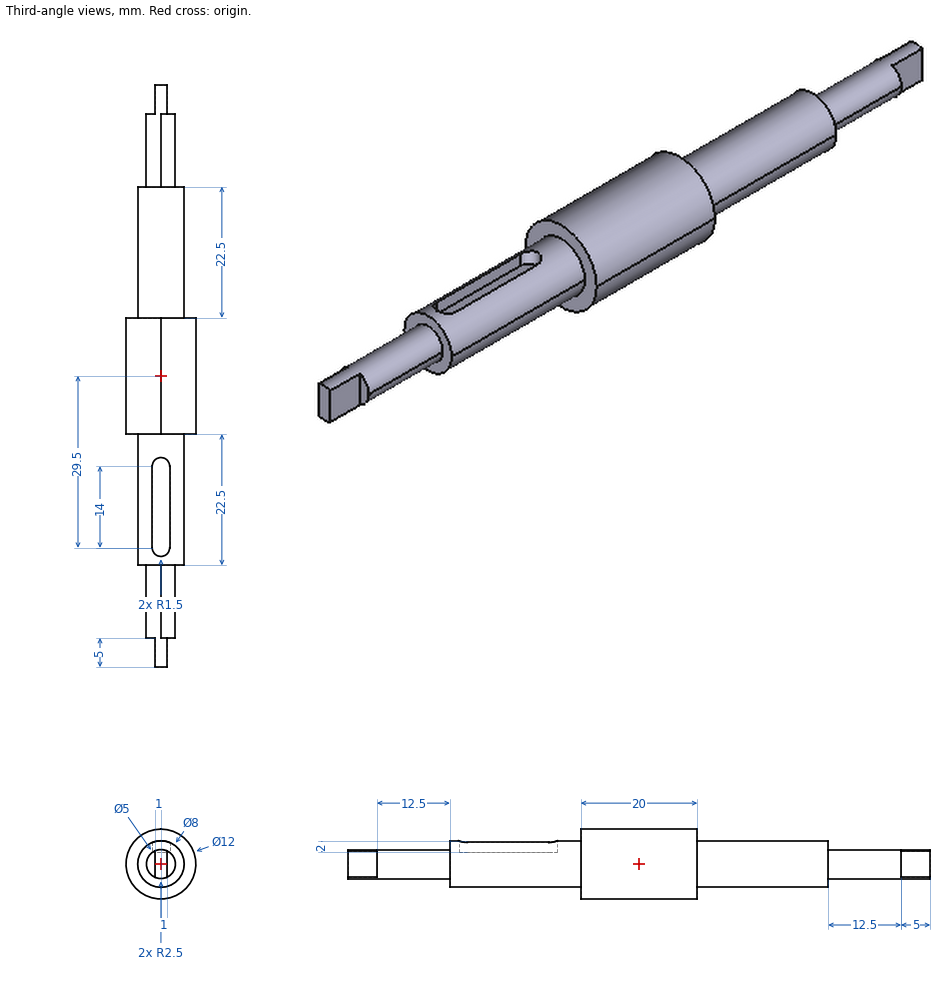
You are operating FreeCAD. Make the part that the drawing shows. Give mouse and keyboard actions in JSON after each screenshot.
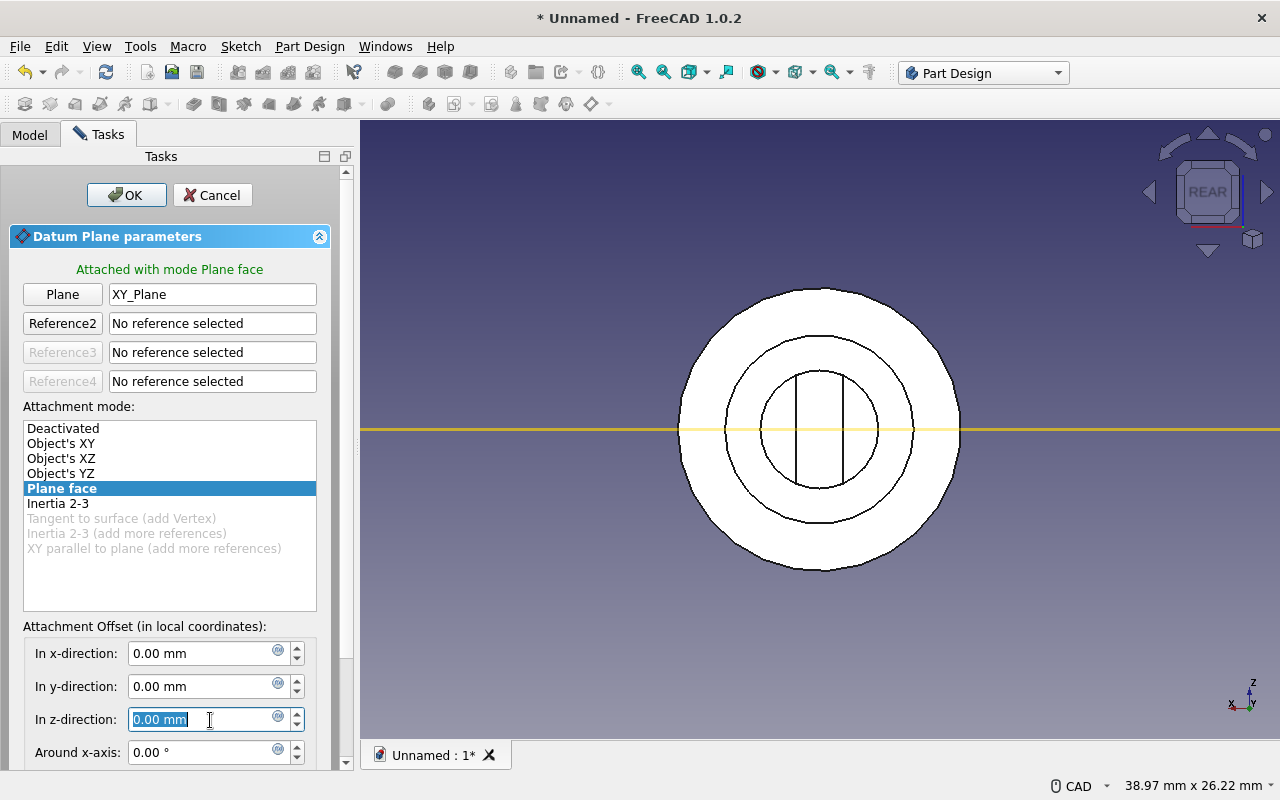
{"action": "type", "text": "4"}
{"action": "key", "text": "Tab"}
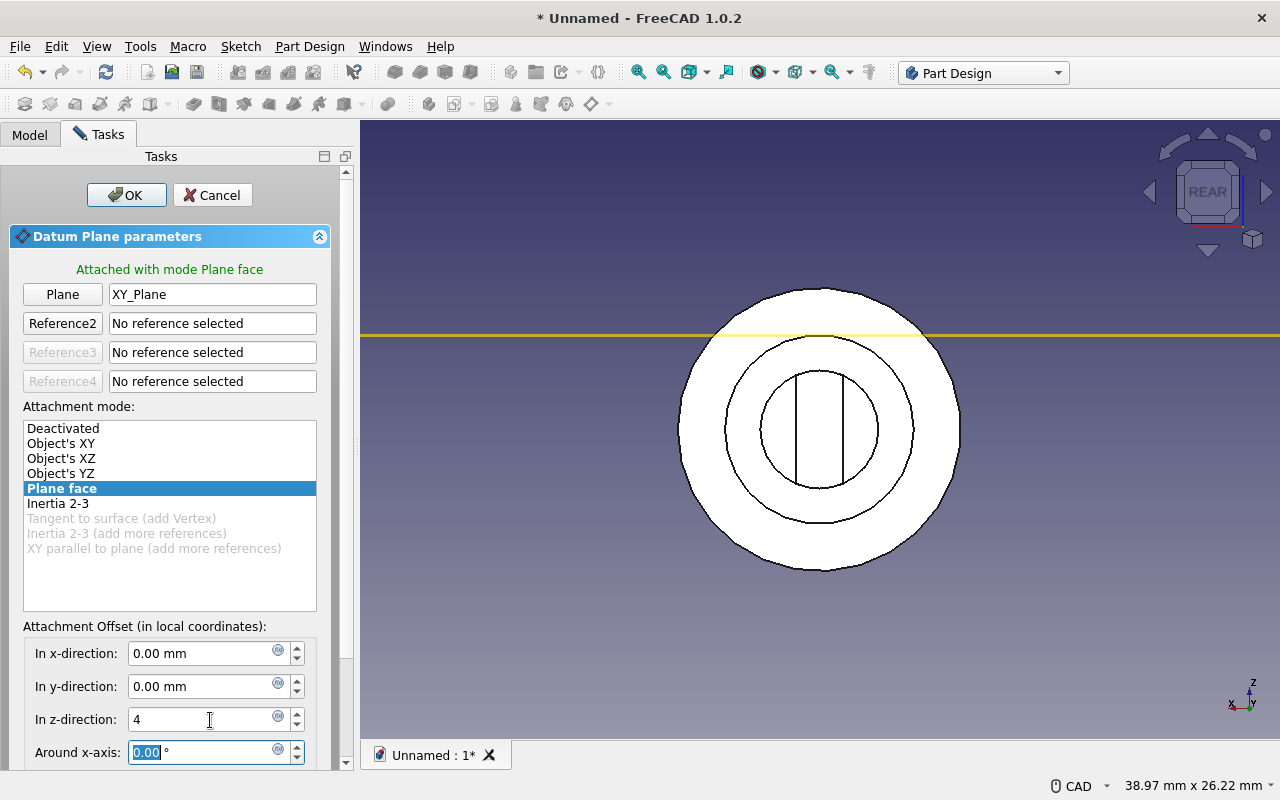
{"action": "left_click", "coordinate": [127, 195]}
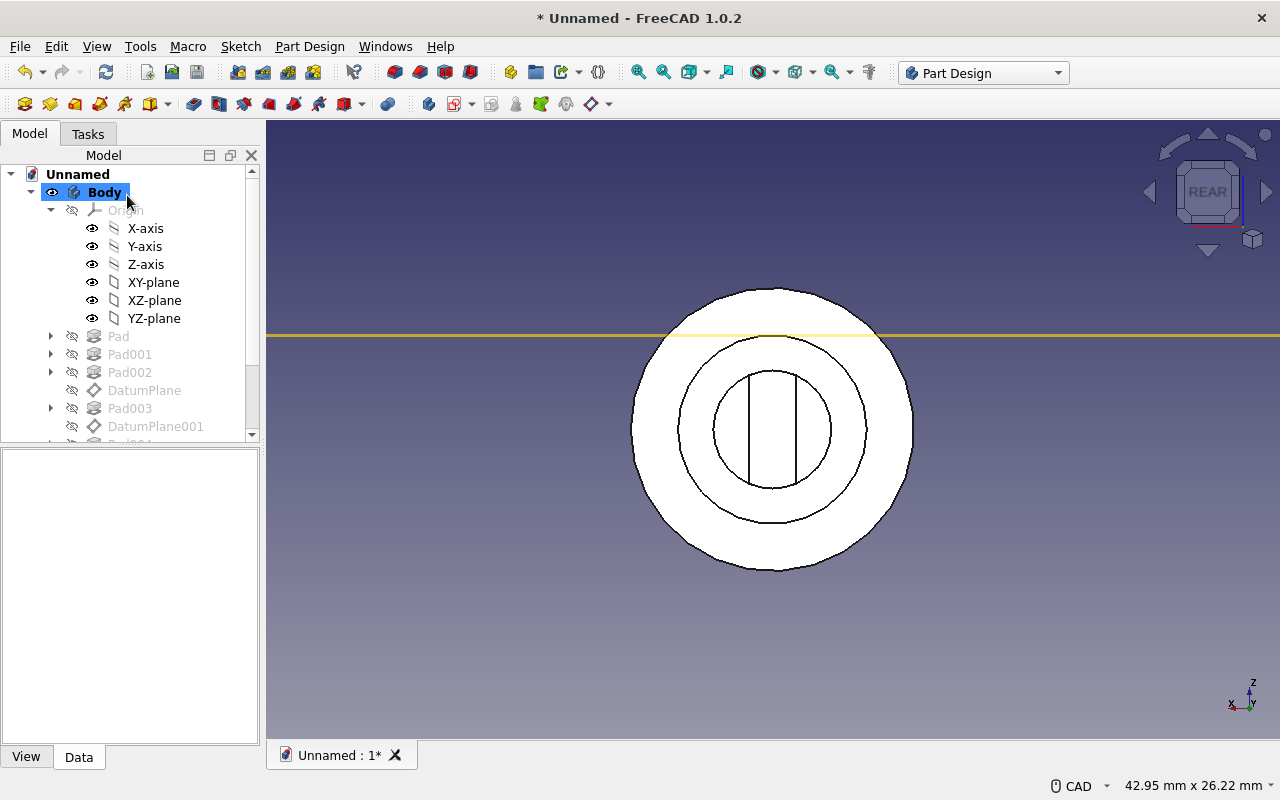
{"action": "scroll", "coordinate": [101, 296], "scroll_direction": "down", "scroll_amount": 3}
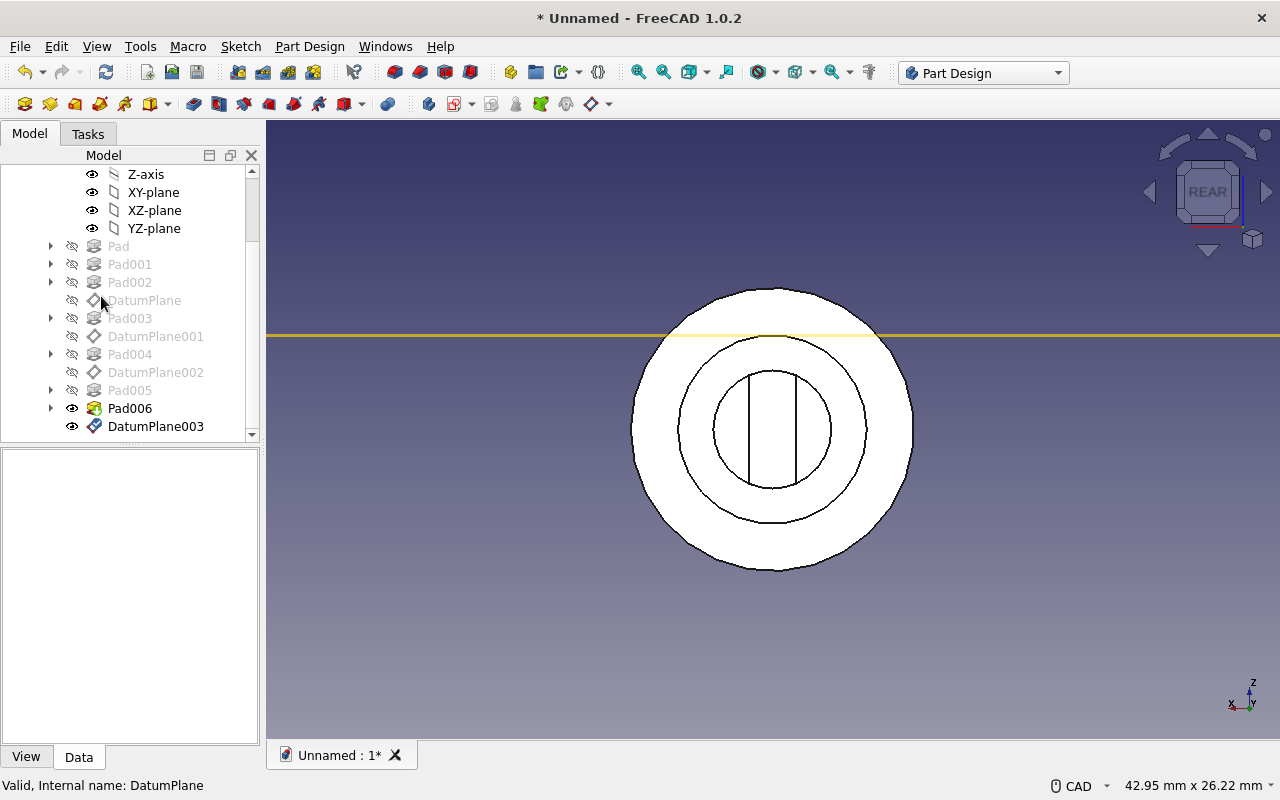
{"action": "left_click", "coordinate": [117, 426]}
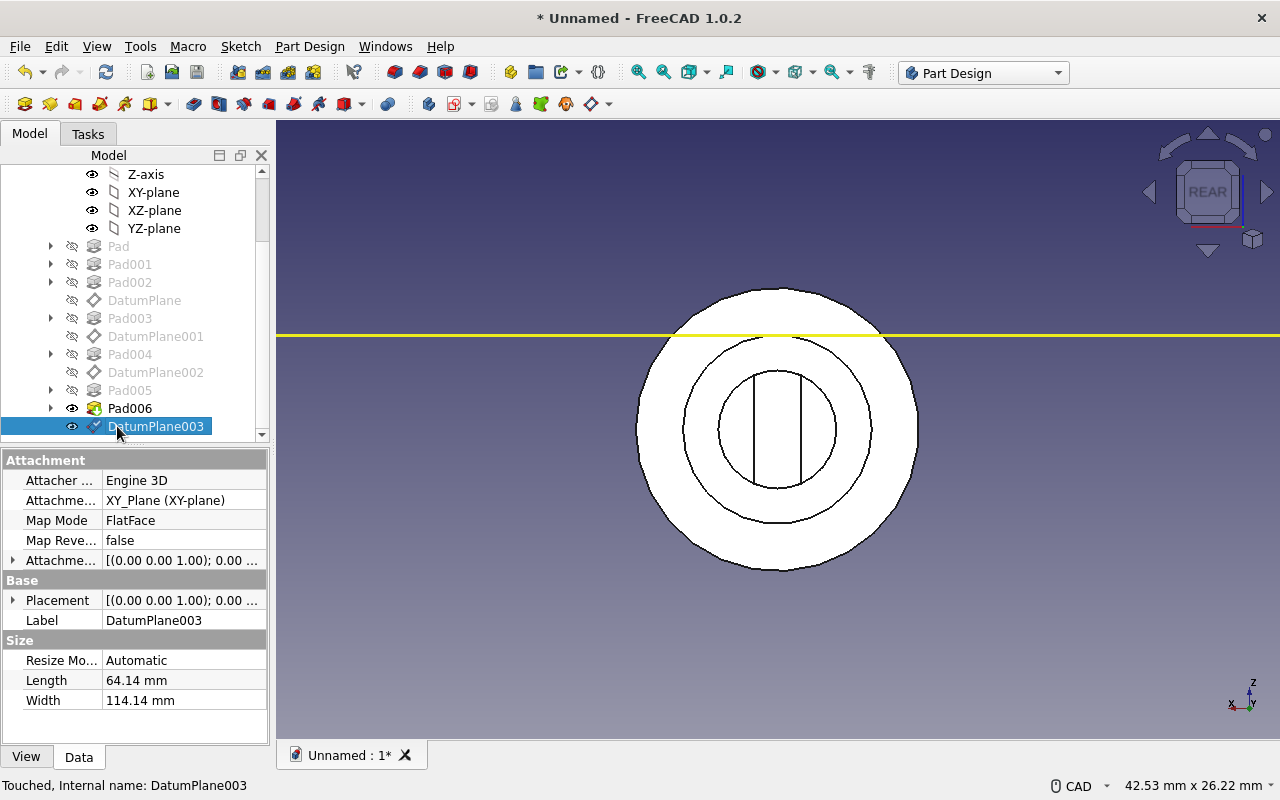
{"action": "left_click", "coordinate": [454, 104]}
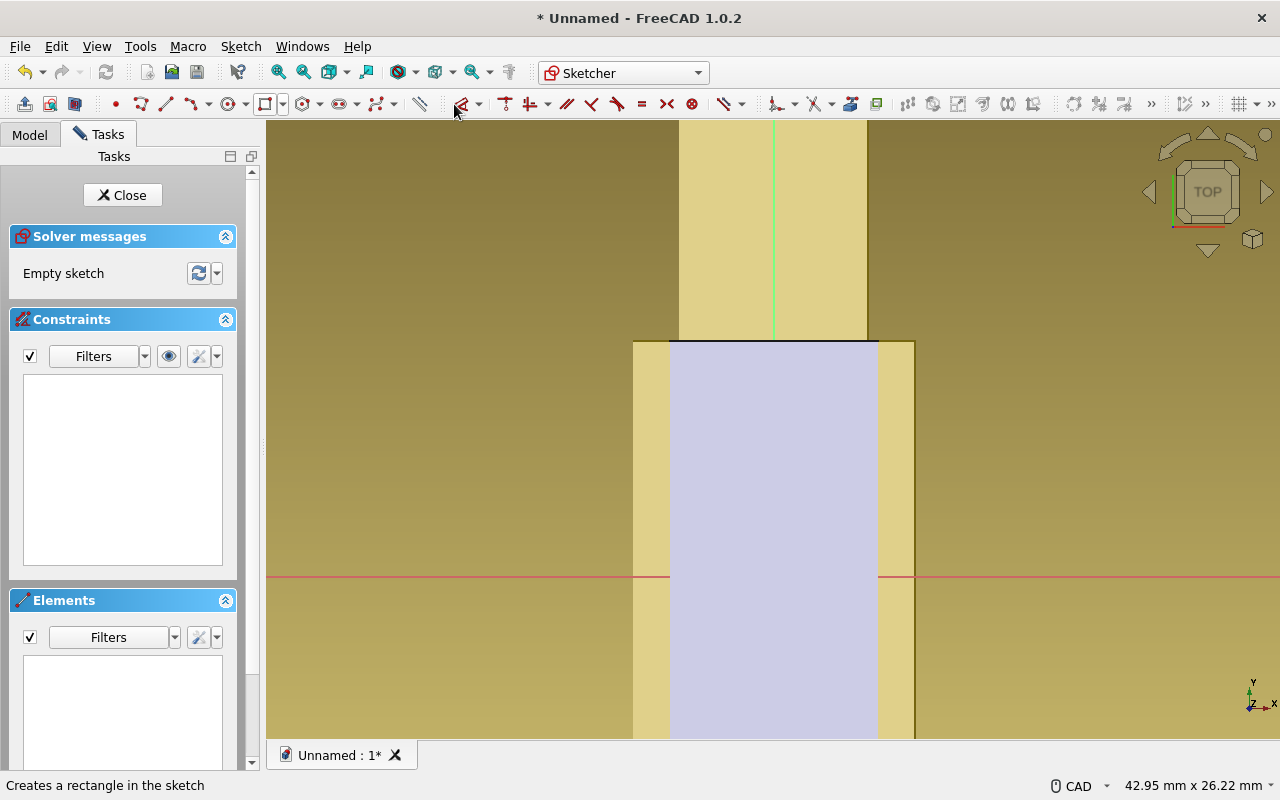
{"action": "left_click", "coordinate": [75, 104]}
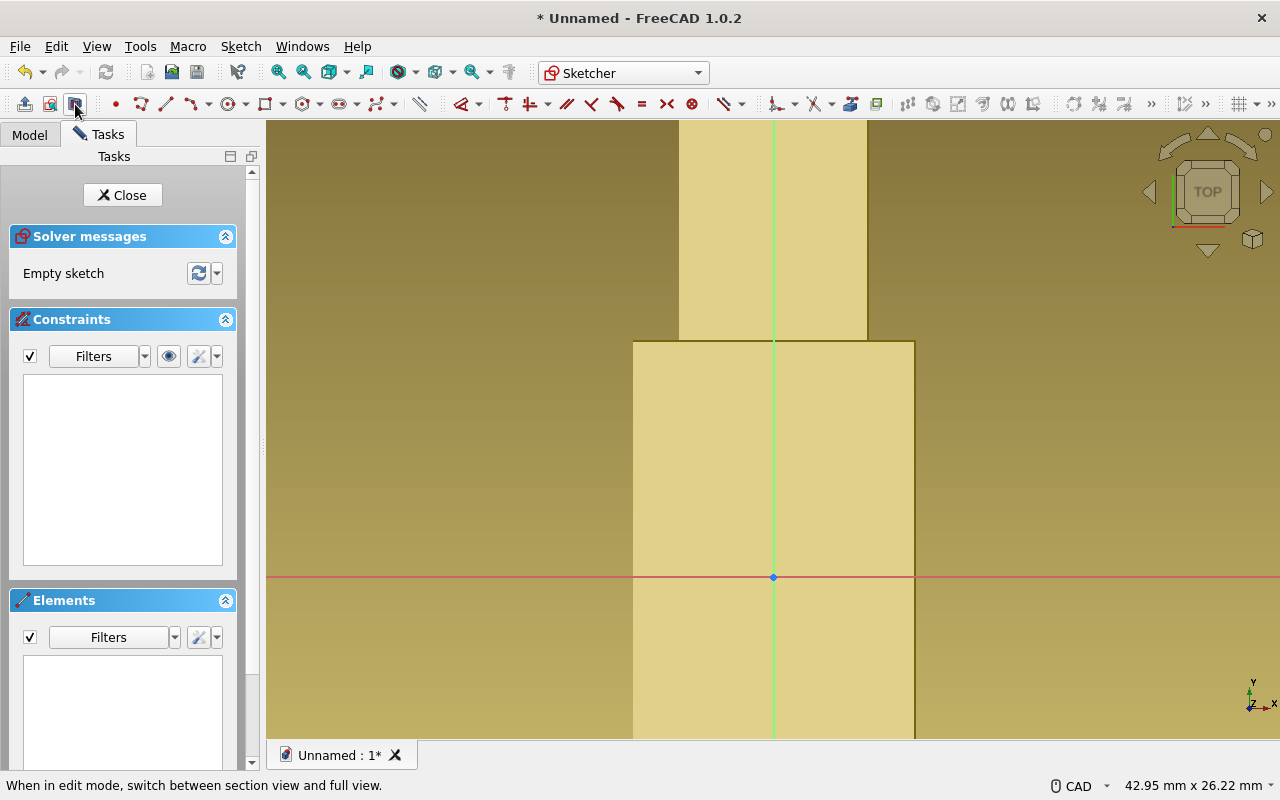
{"action": "scroll", "coordinate": [648, 148], "scroll_direction": "down", "scroll_amount": 4}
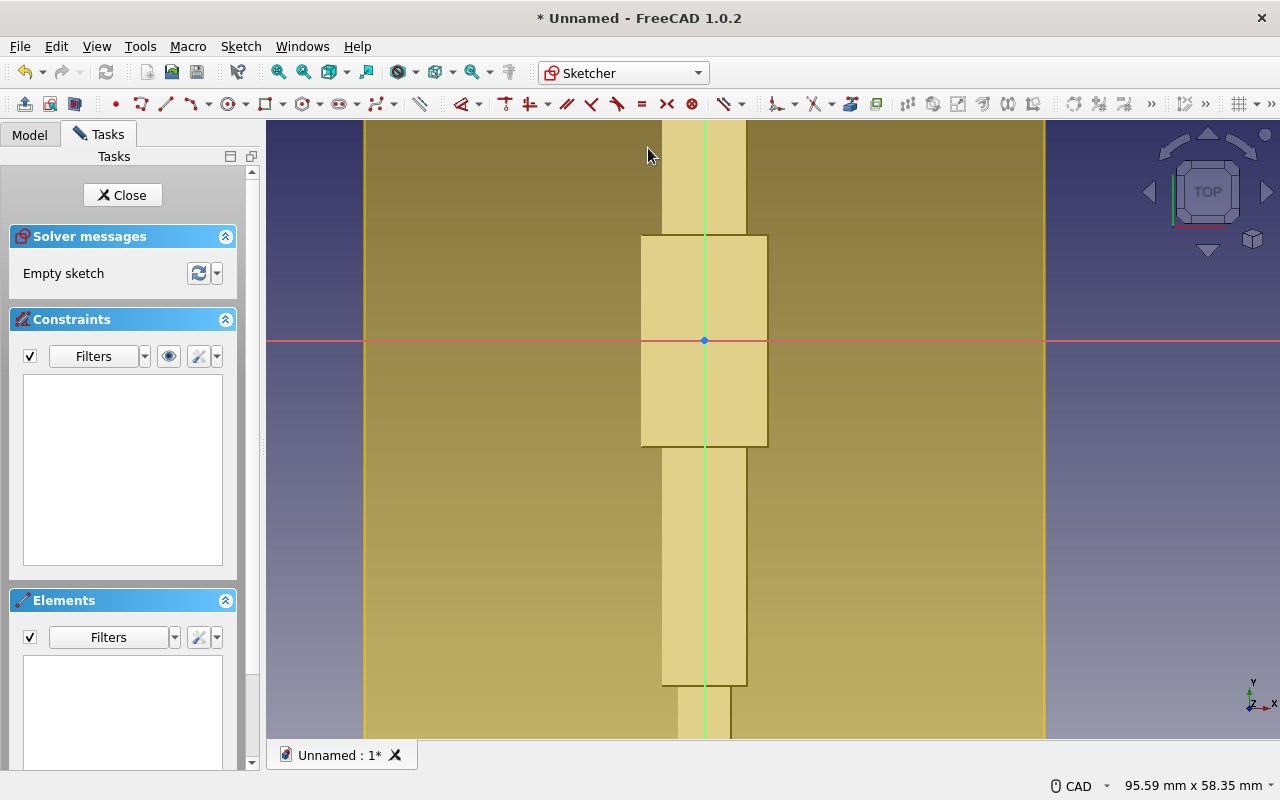
{"action": "key", "text": "g s"}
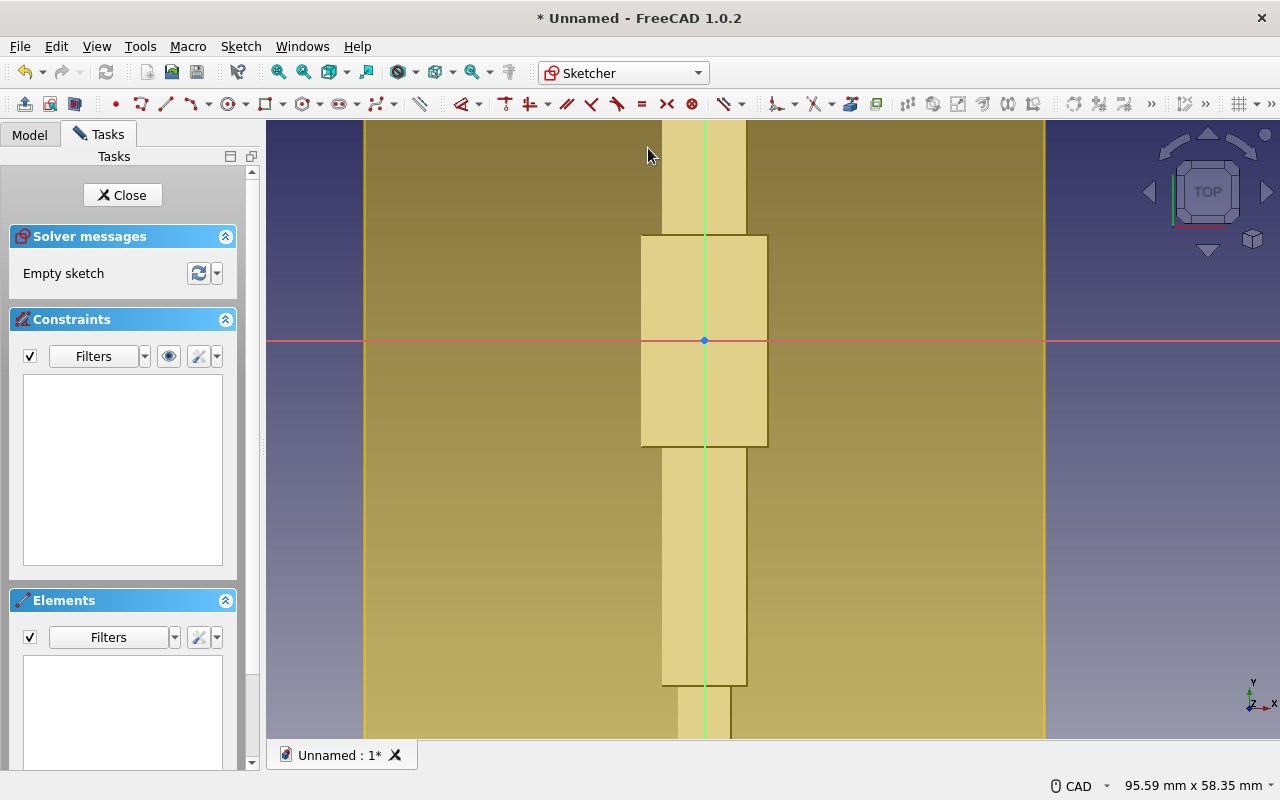
{"action": "scroll", "coordinate": [705, 654], "scroll_direction": "up", "scroll_amount": 2}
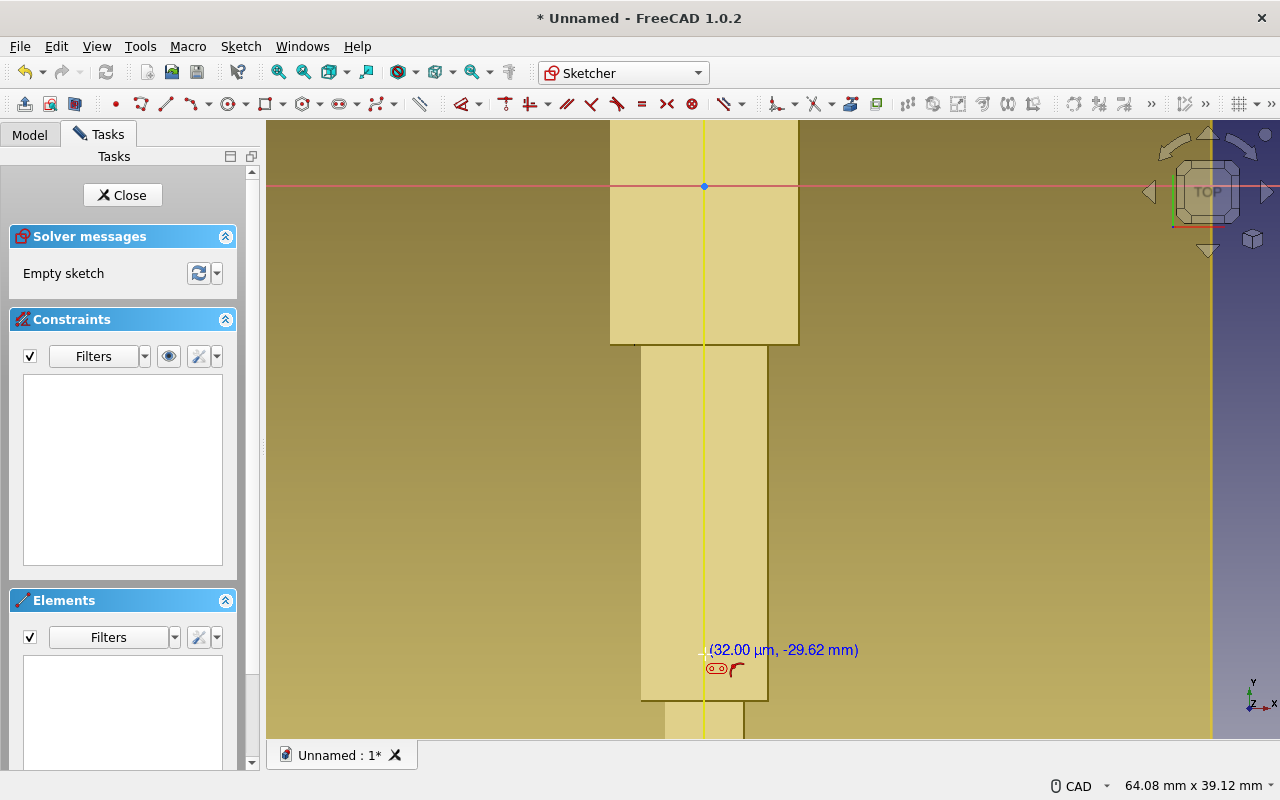
{"action": "left_click", "coordinate": [704, 653]}